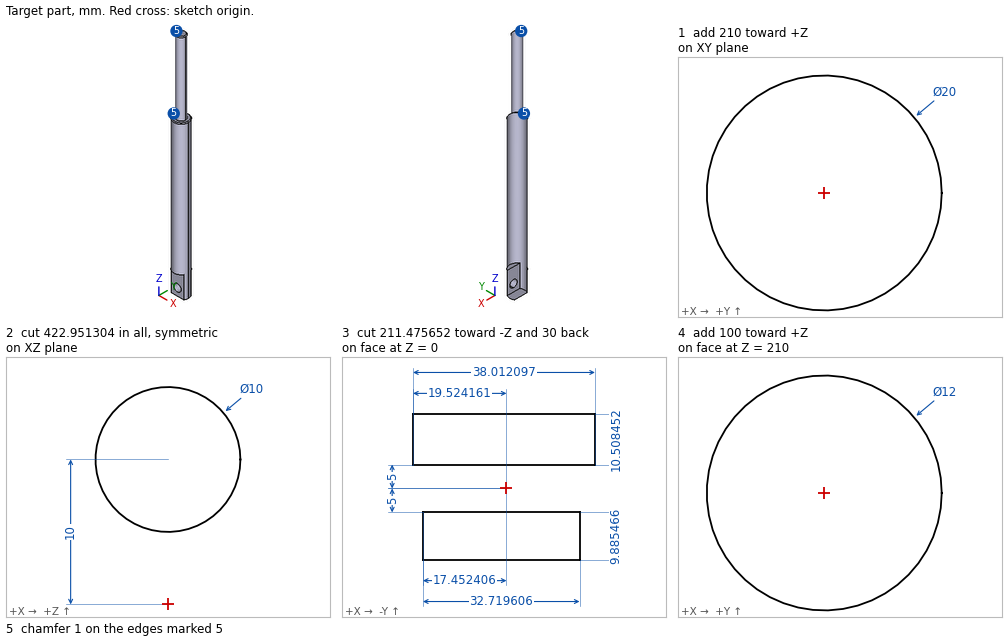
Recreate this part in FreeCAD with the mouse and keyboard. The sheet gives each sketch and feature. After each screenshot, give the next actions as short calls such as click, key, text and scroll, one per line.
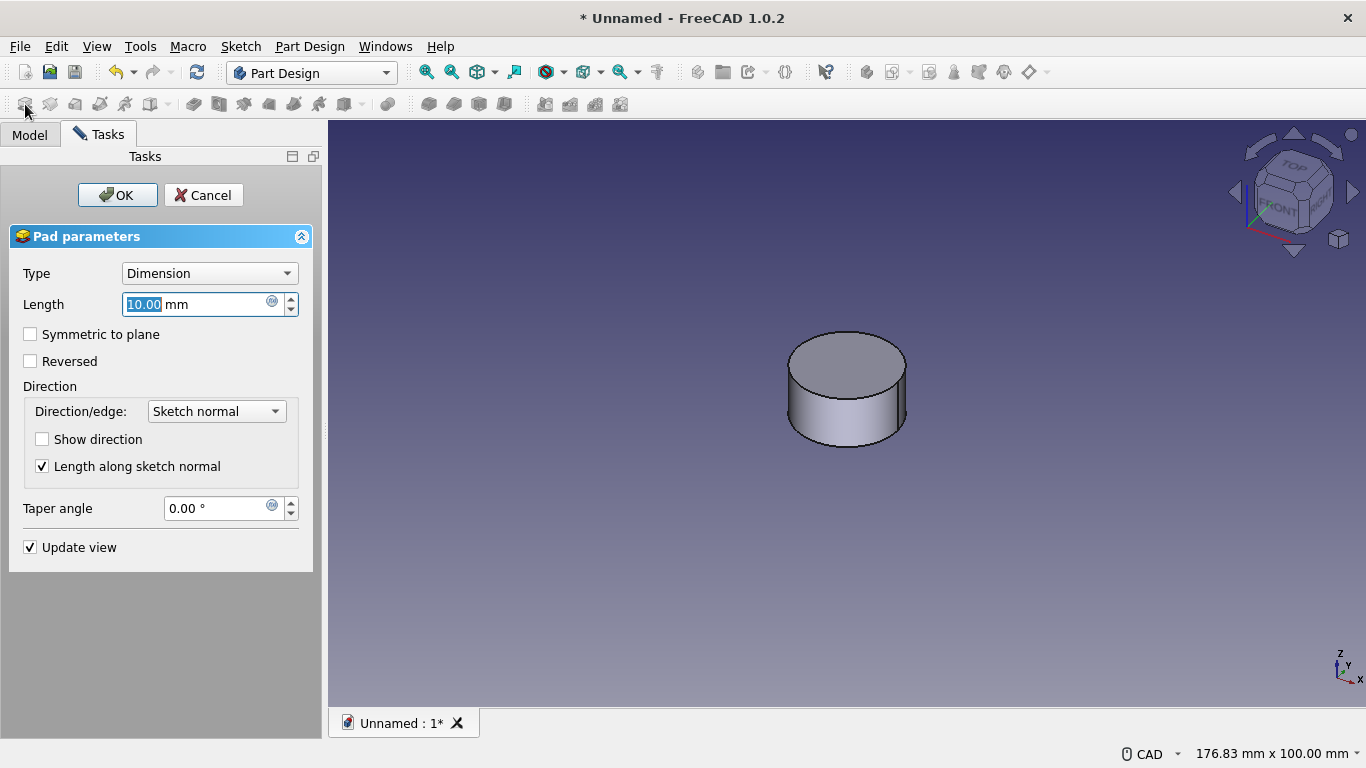
text(210)
key(Tab)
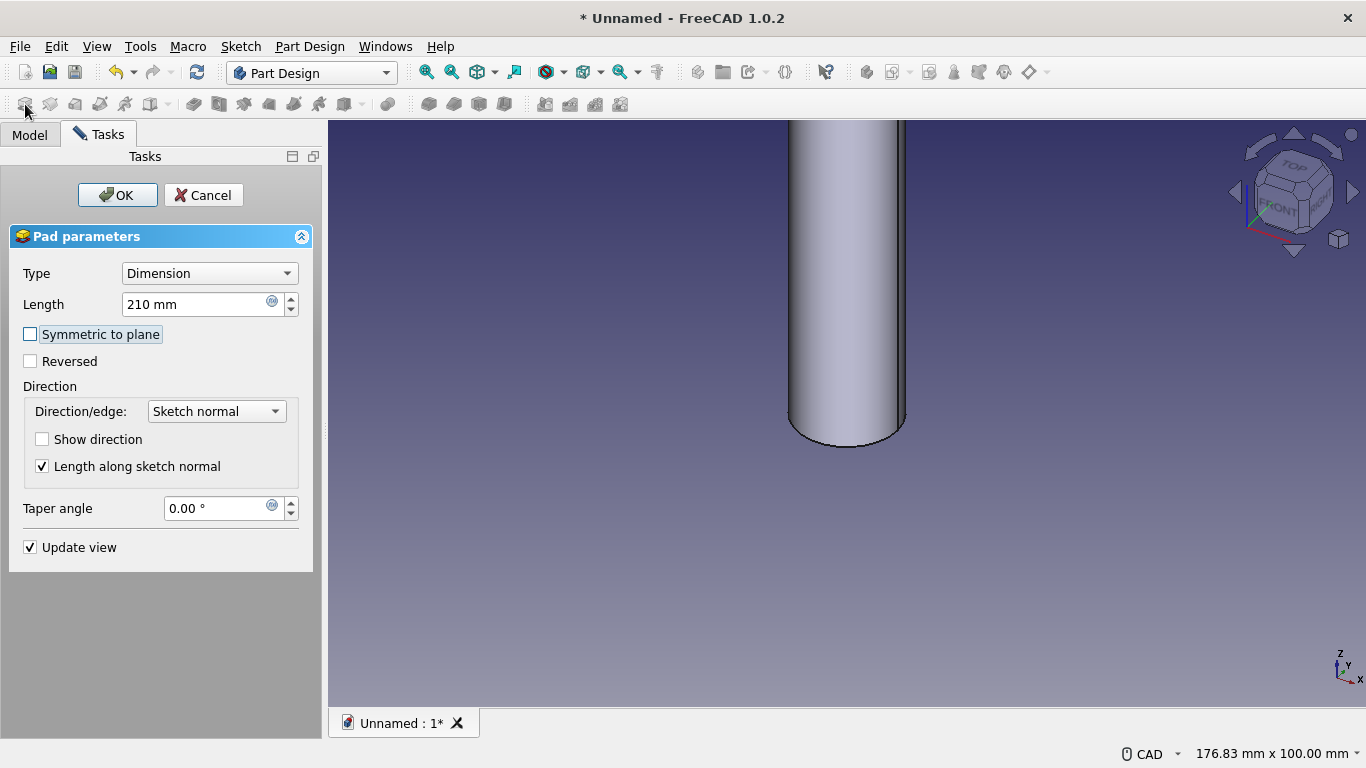
click(118, 195)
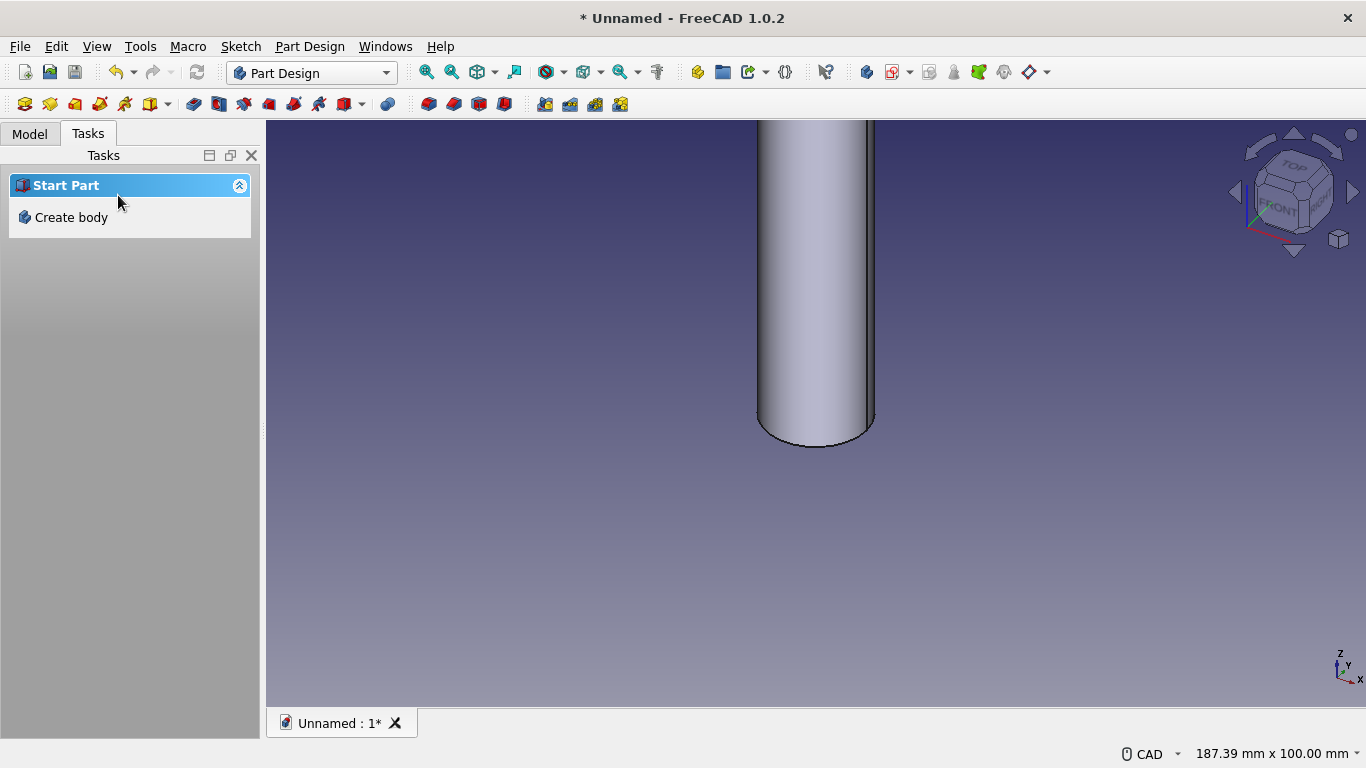
click(427, 72)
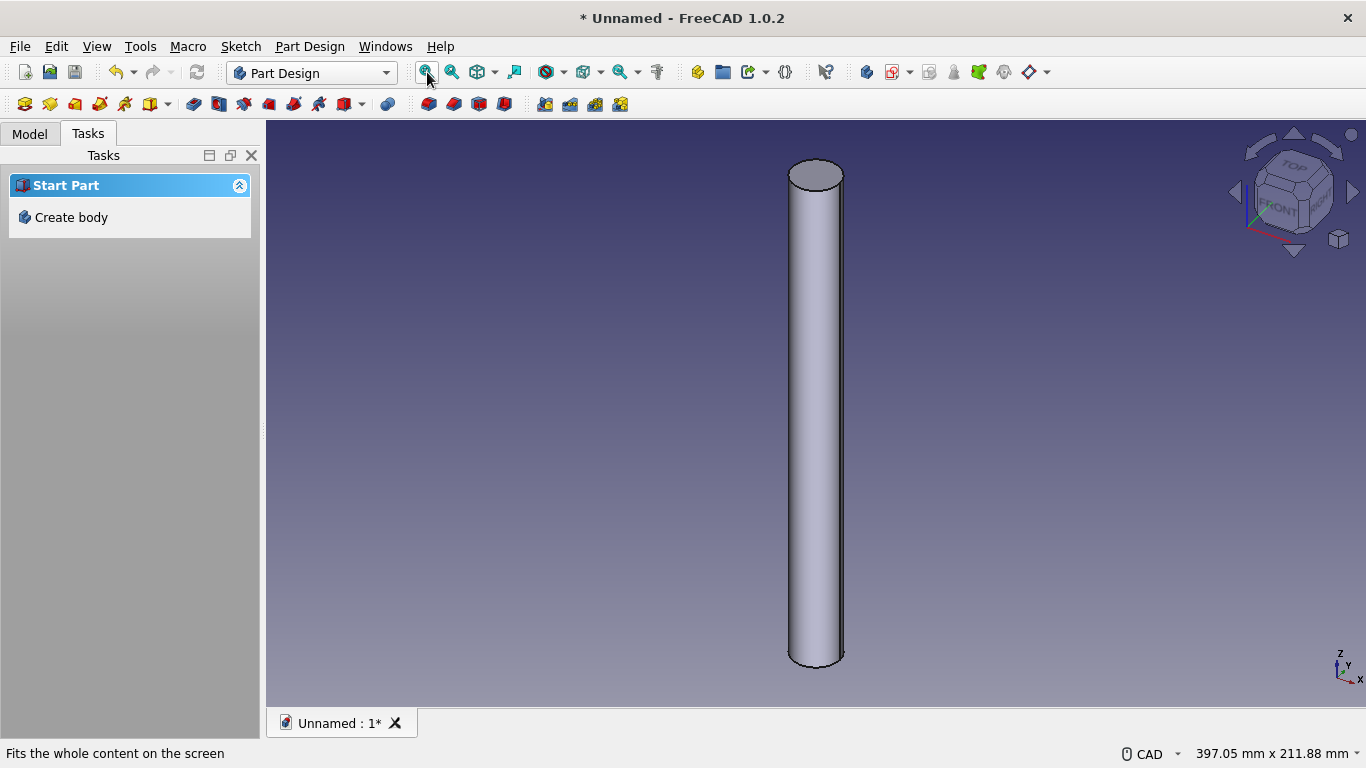
click(892, 72)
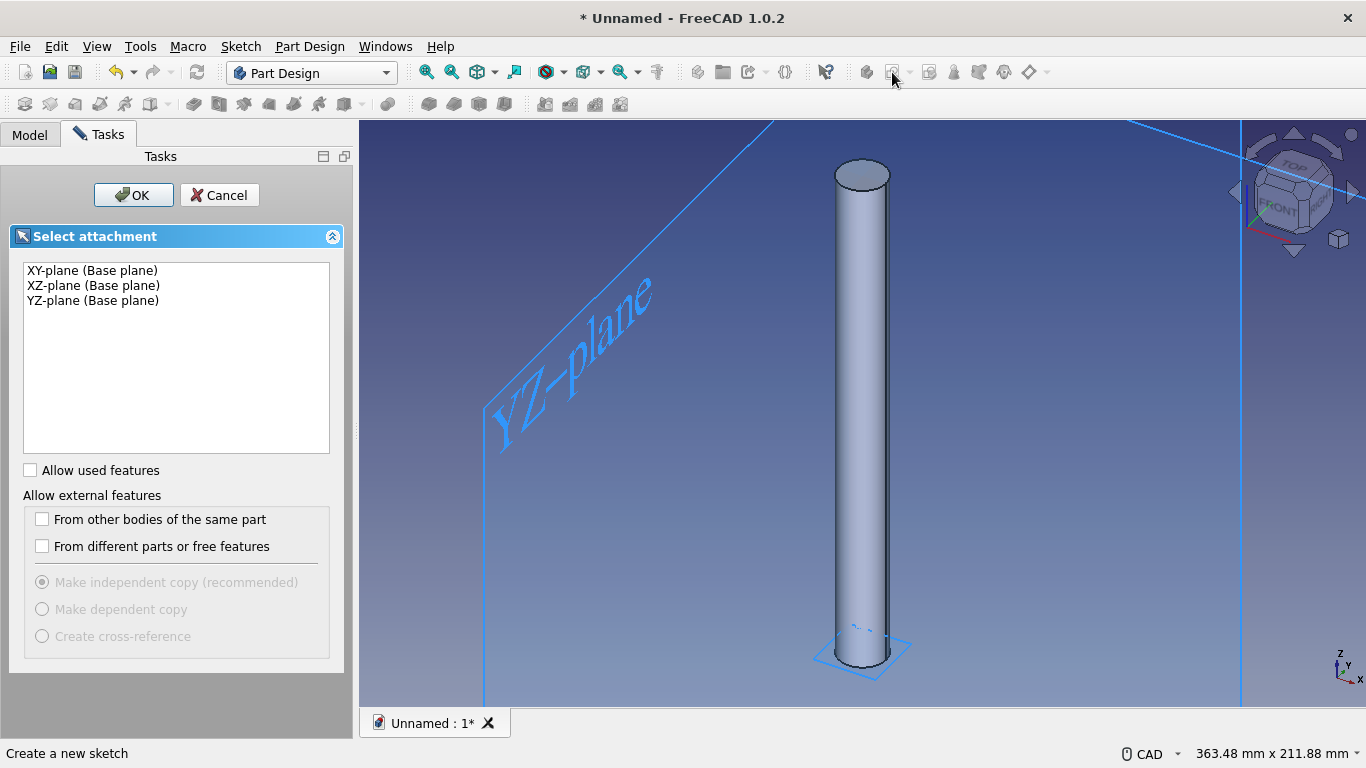
click(84, 286)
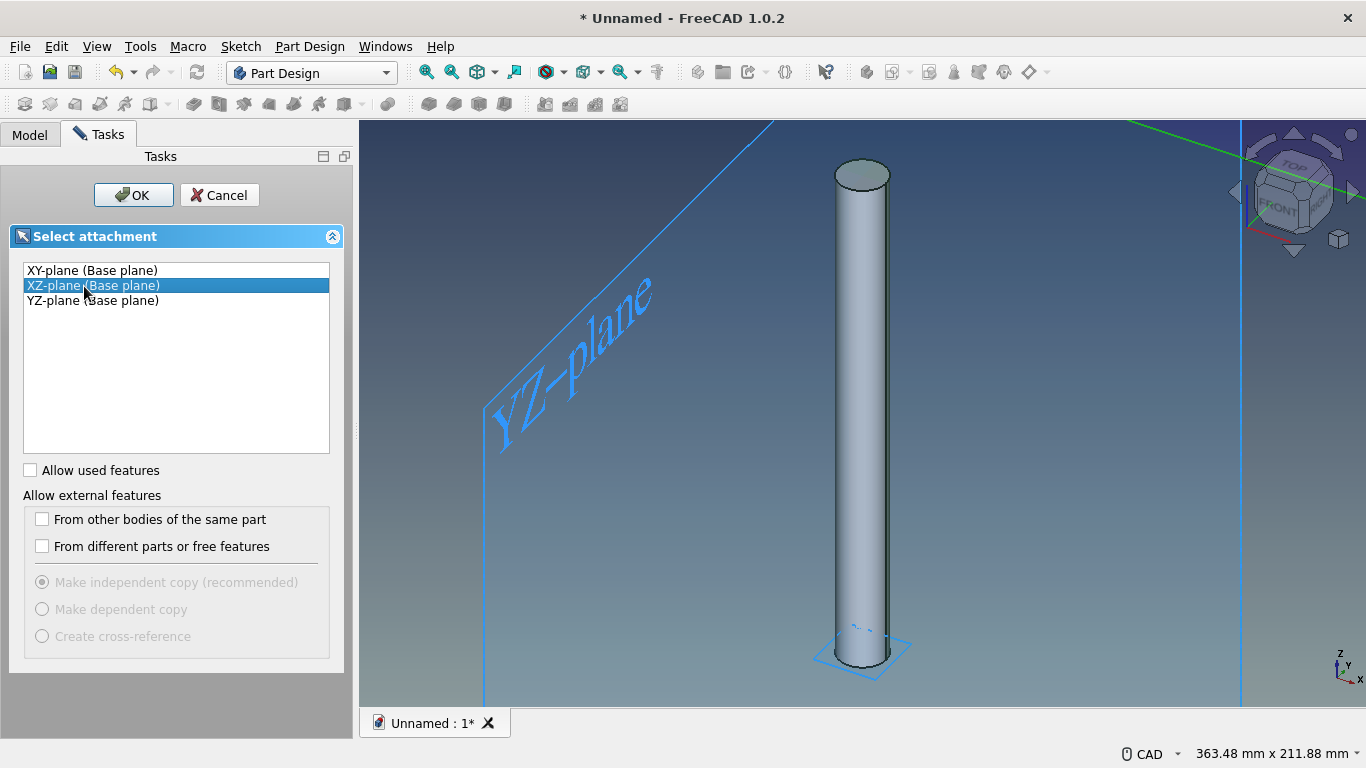
click(134, 195)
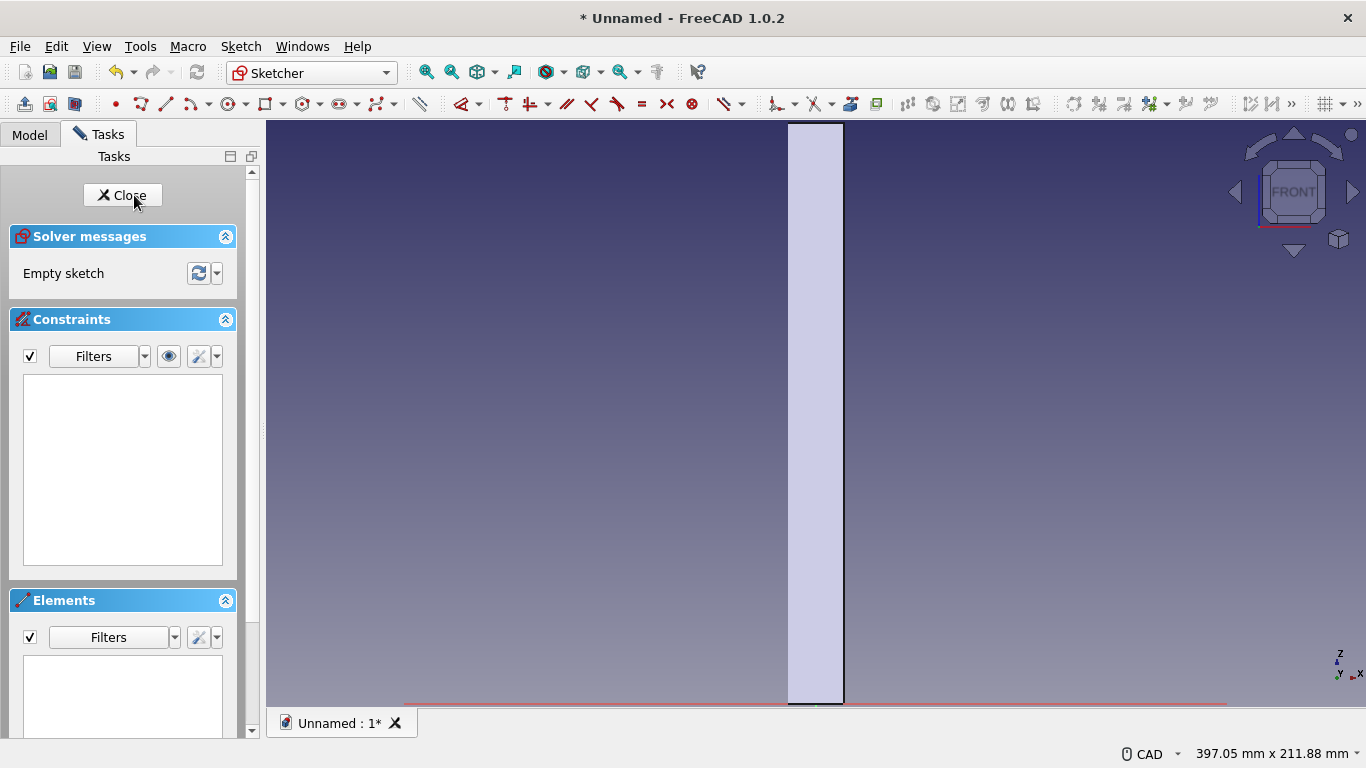
click(75, 104)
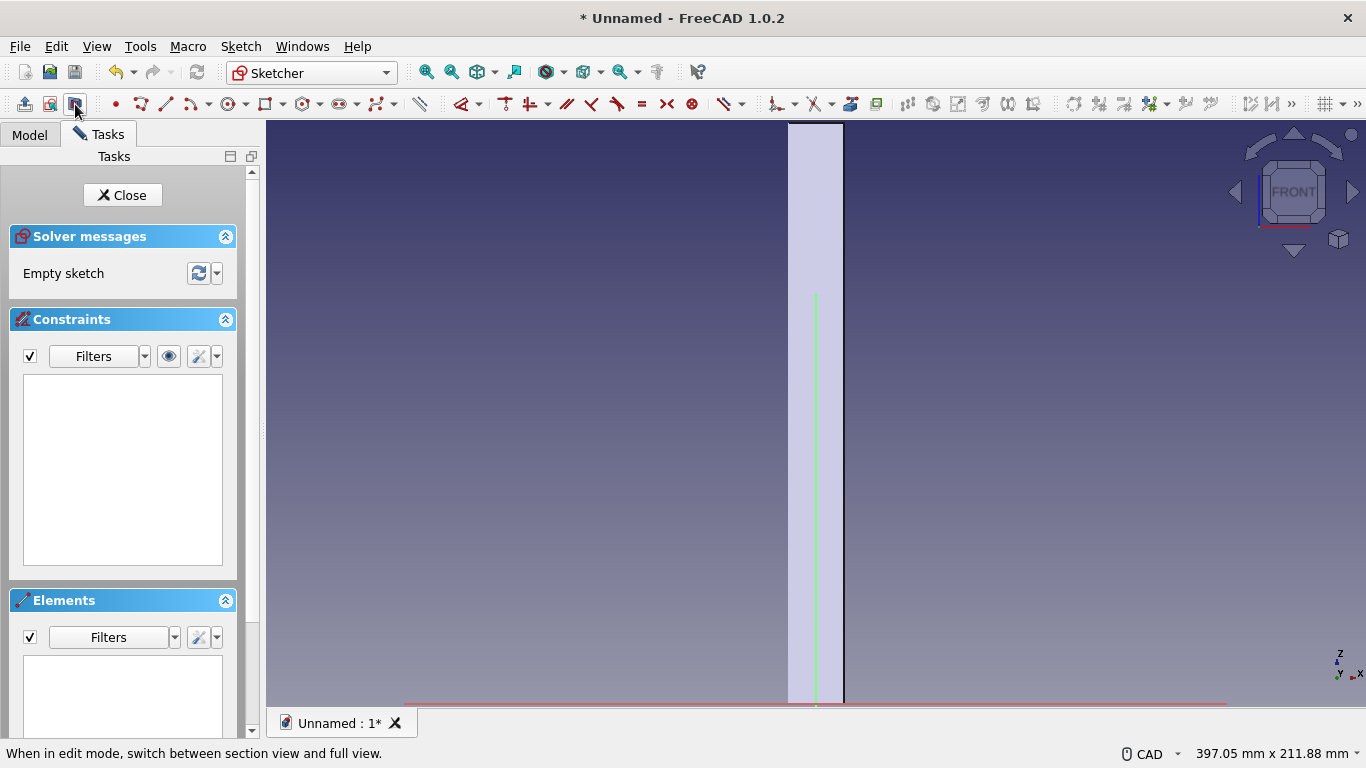
scroll(748, 414, down, 5)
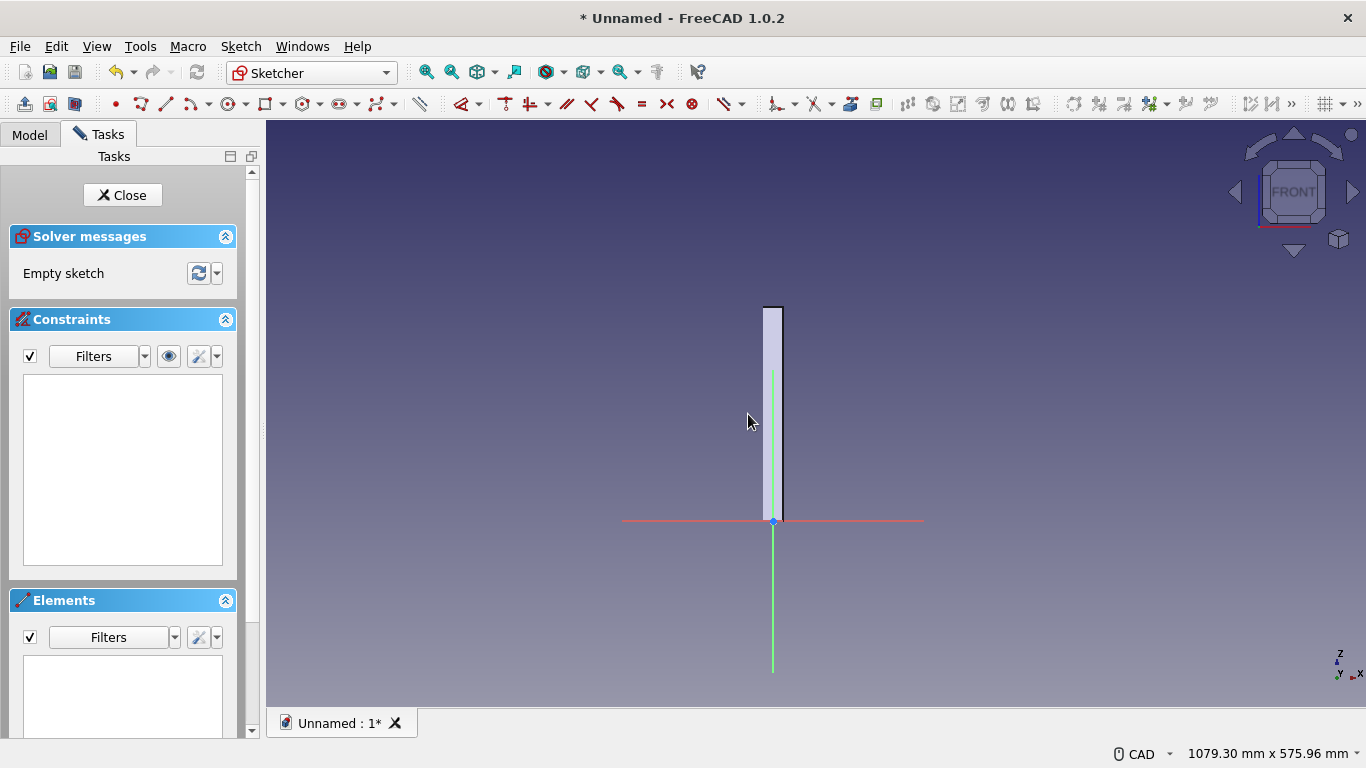
scroll(775, 519, up, 15)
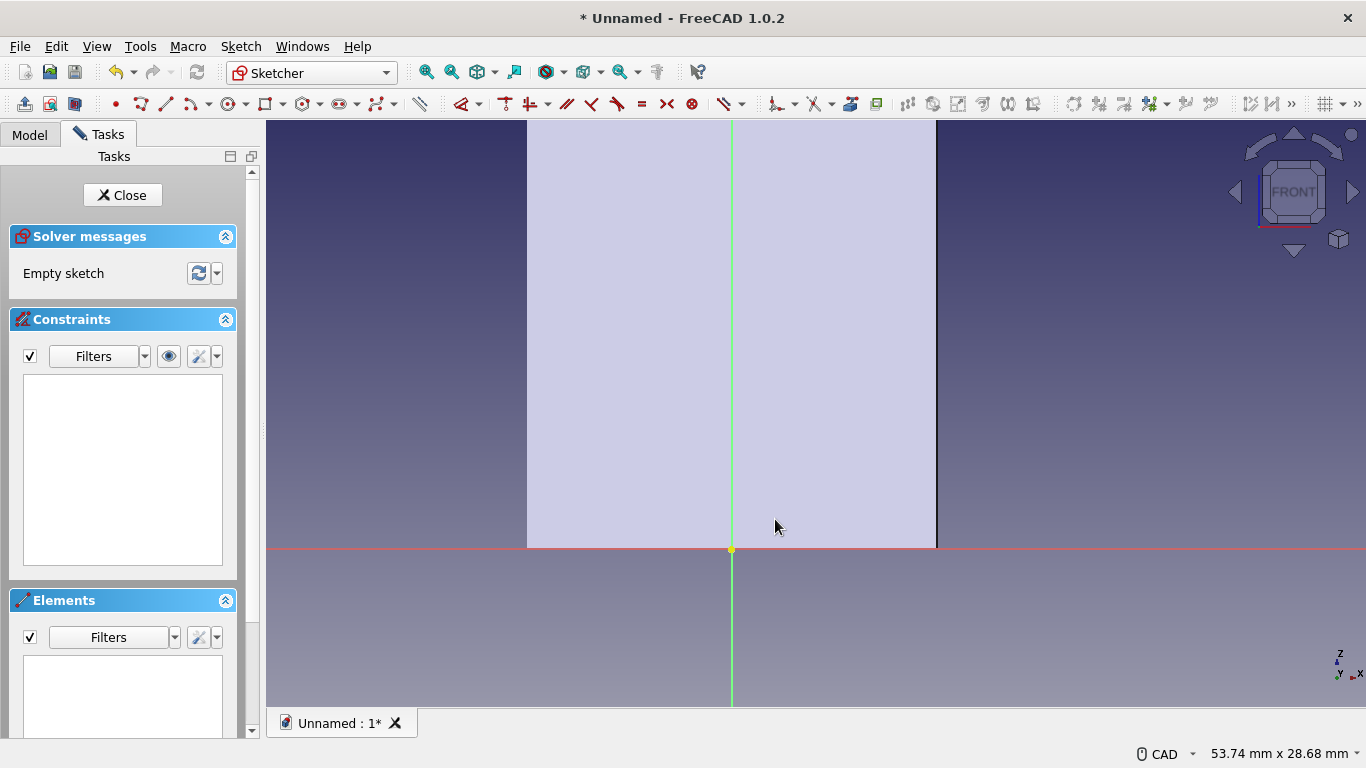
key(g)
key(c)